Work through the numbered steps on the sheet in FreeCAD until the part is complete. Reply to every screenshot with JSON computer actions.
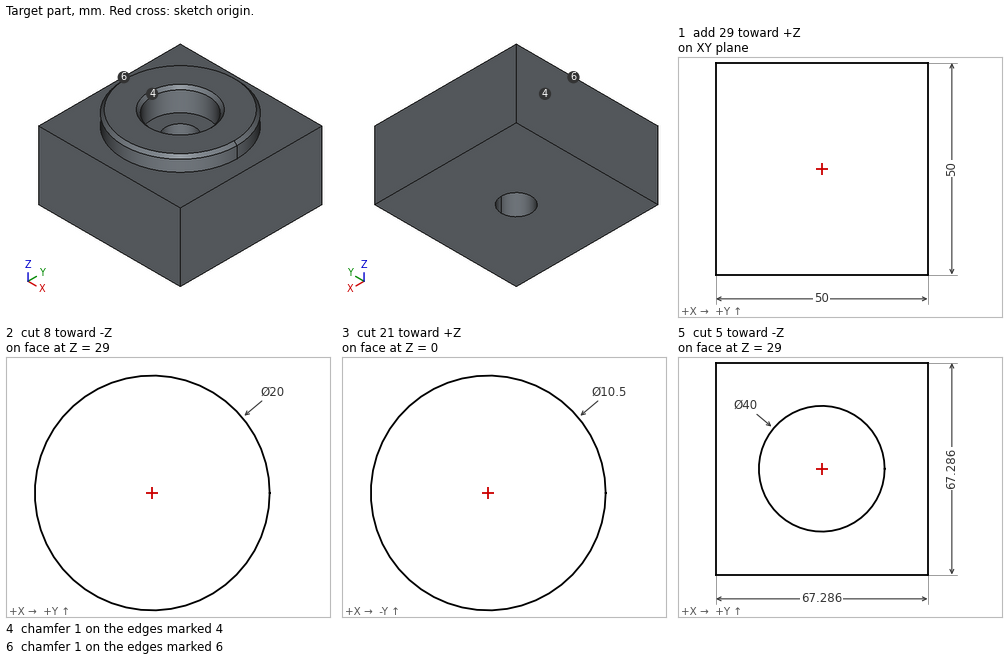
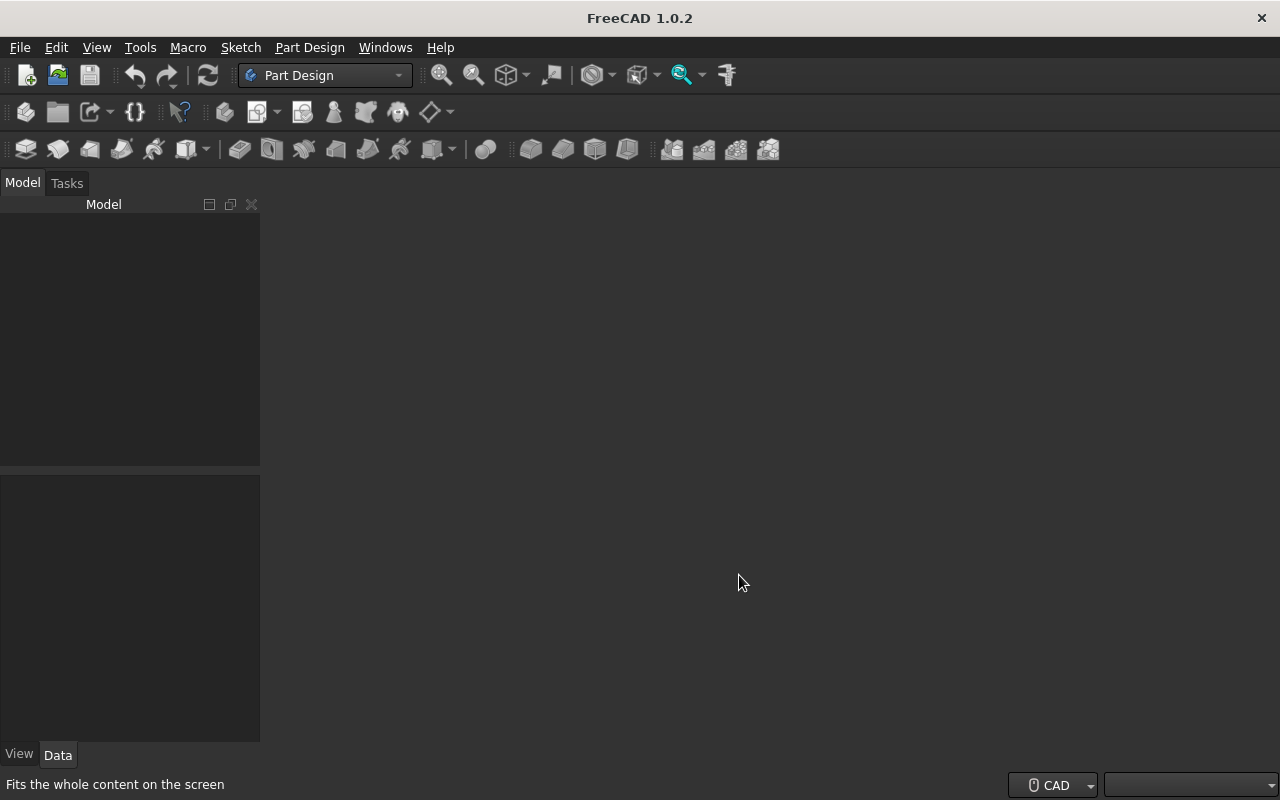
{"action": "left_click", "coordinate": [26, 76]}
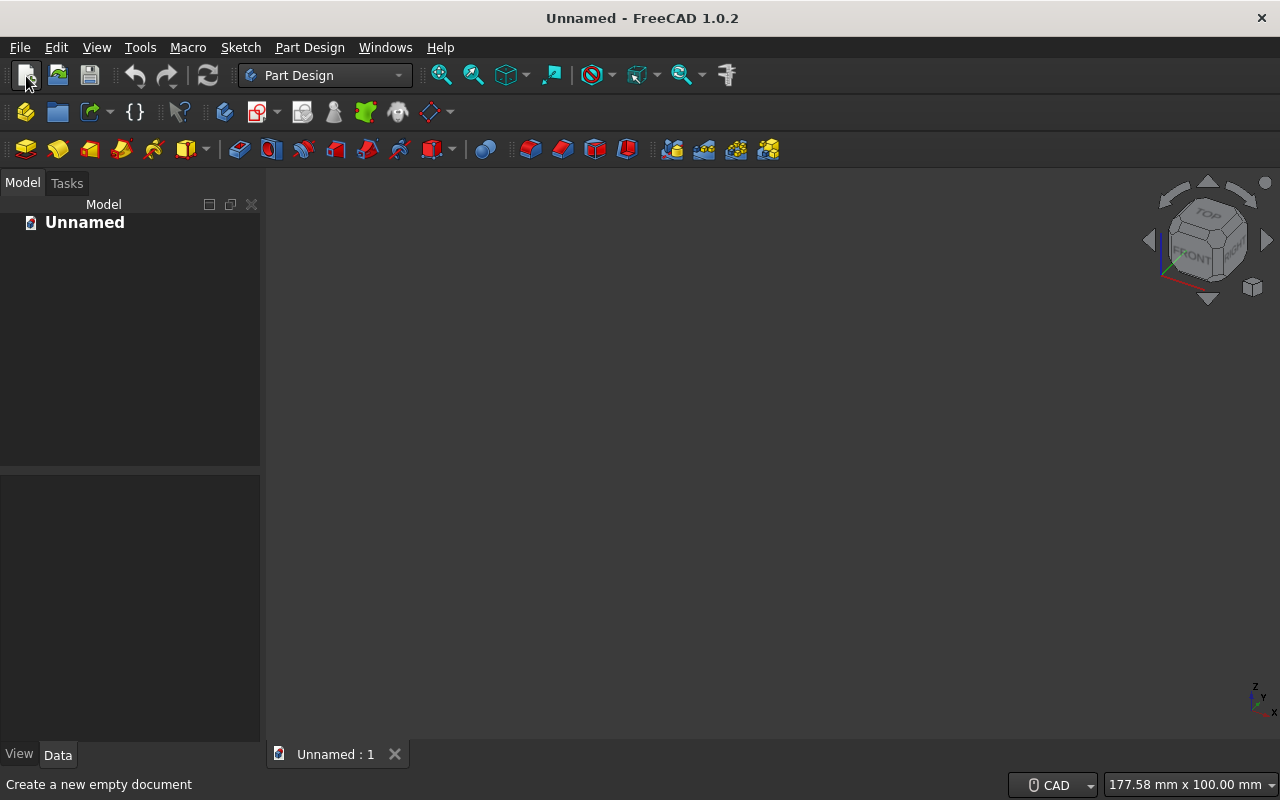
{"action": "left_click", "coordinate": [258, 112]}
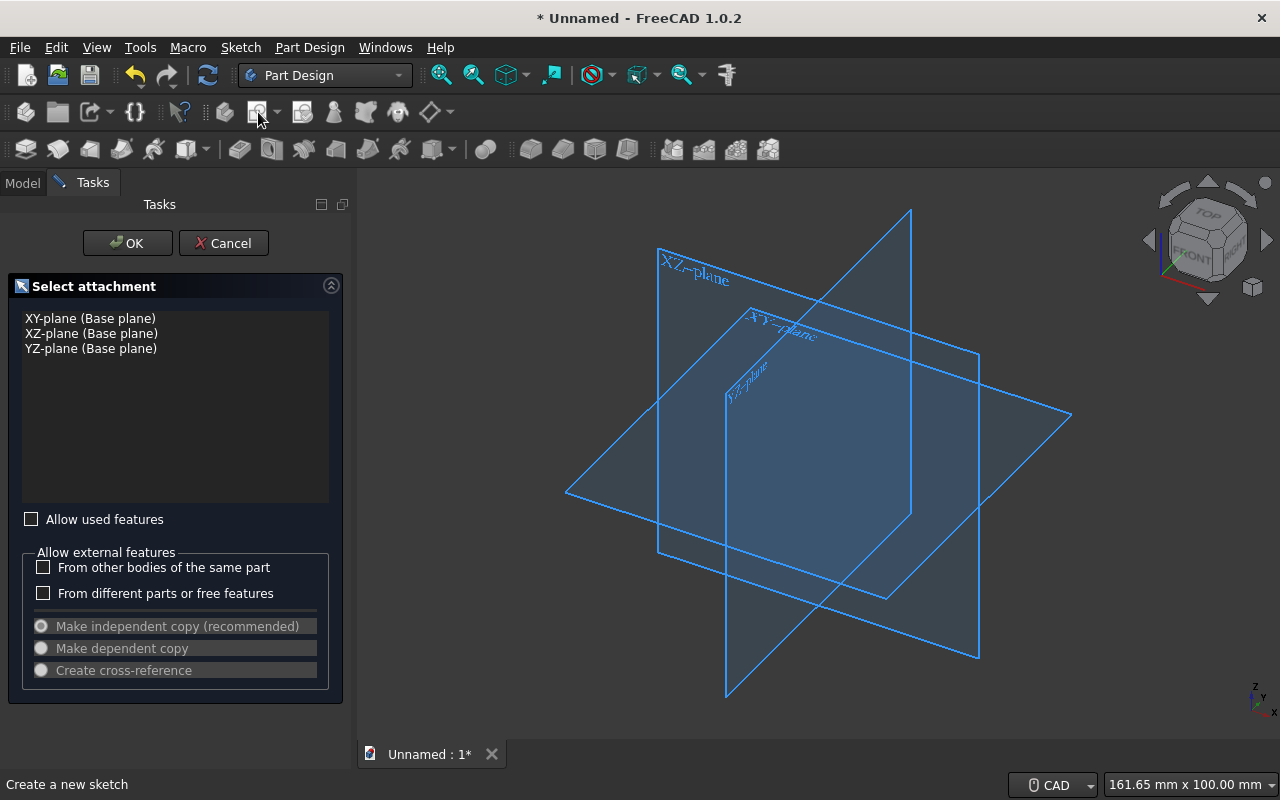
{"action": "left_click", "coordinate": [82, 318]}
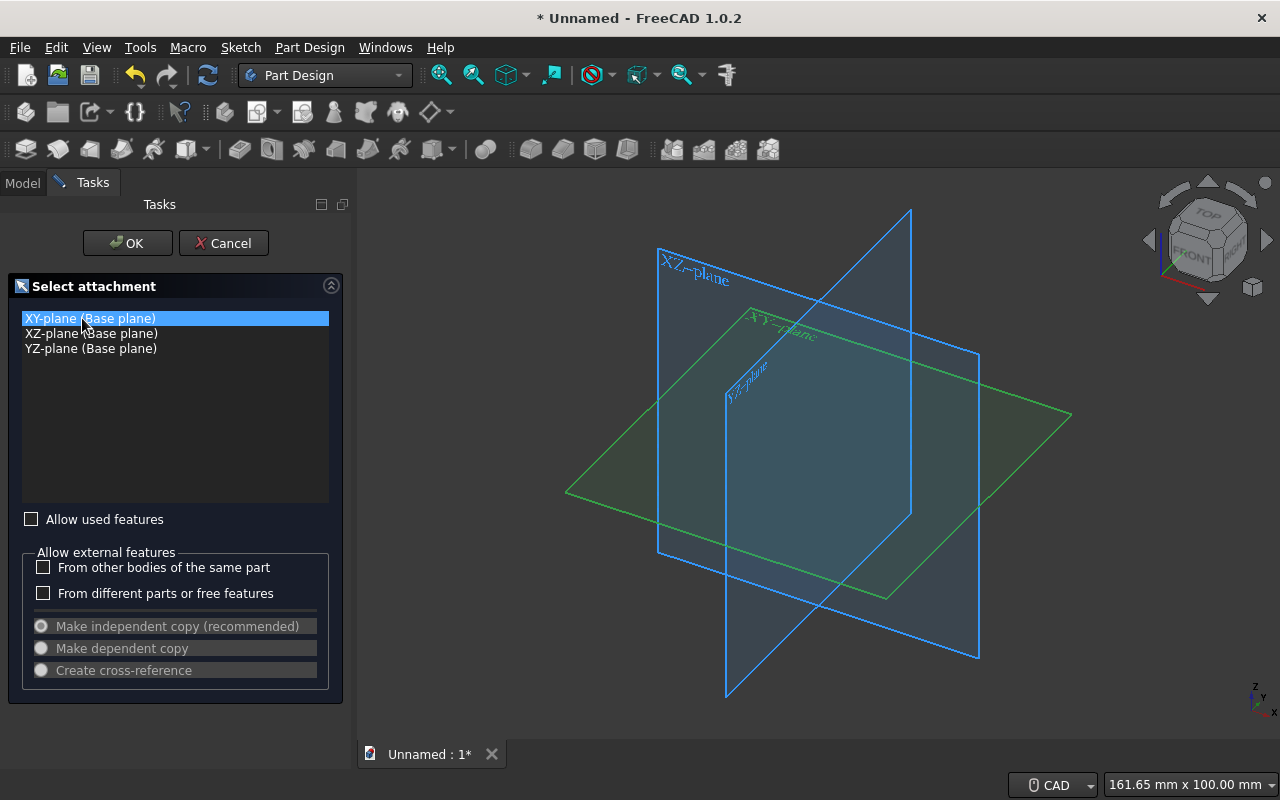
{"action": "left_click", "coordinate": [128, 243]}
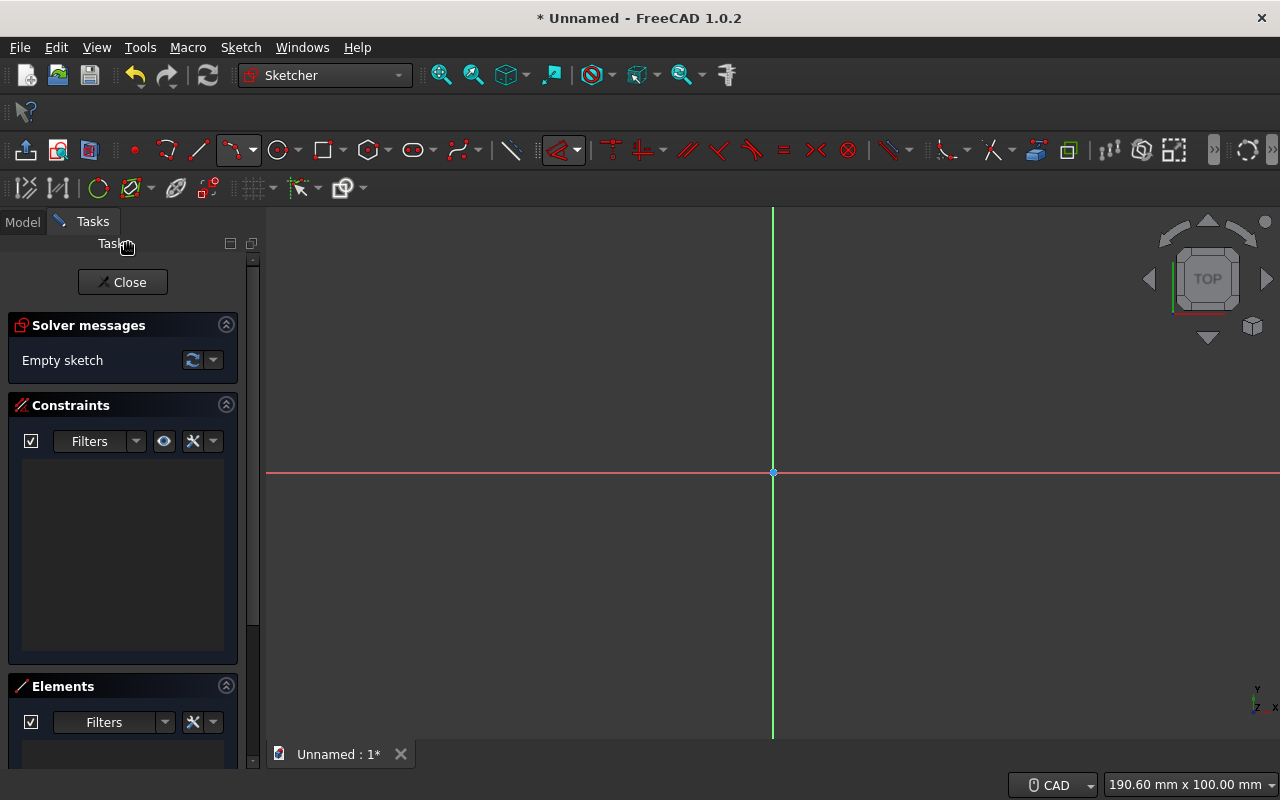
{"action": "key", "text": "g v"}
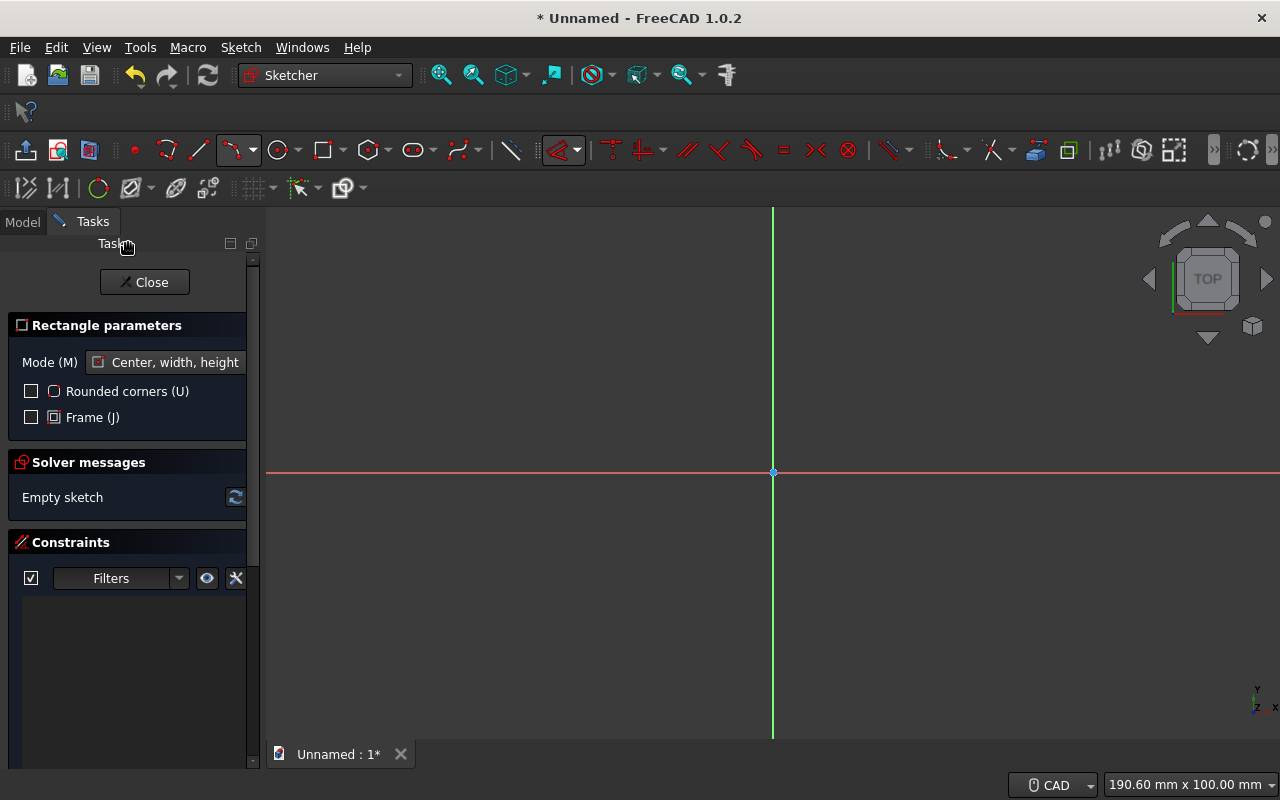
{"action": "left_click", "coordinate": [773, 473]}
{"action": "mouse_move", "coordinate": [906, 340]}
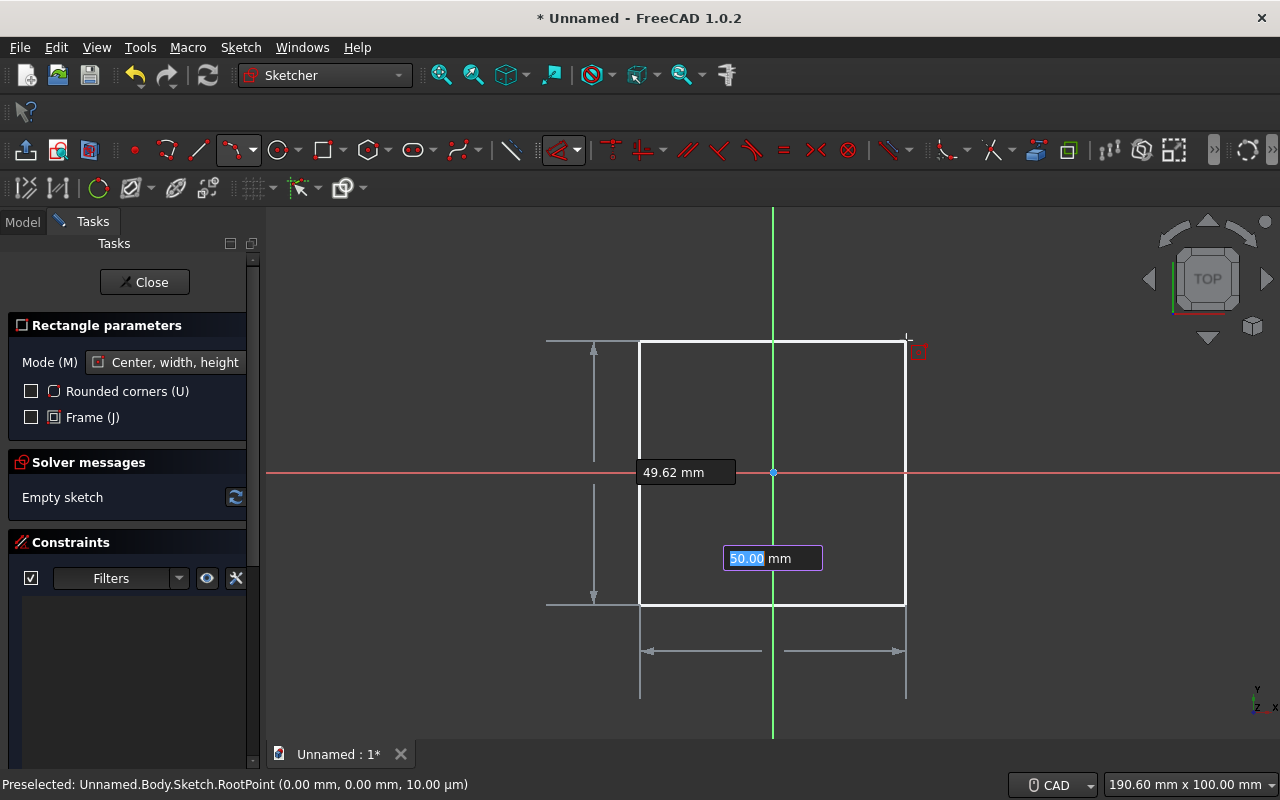
{"action": "type", "text": "50"}
{"action": "key", "text": "Tab"}
{"action": "type", "text": "50"}
{"action": "key", "text": "Return"}
{"action": "key", "text": "Escape"}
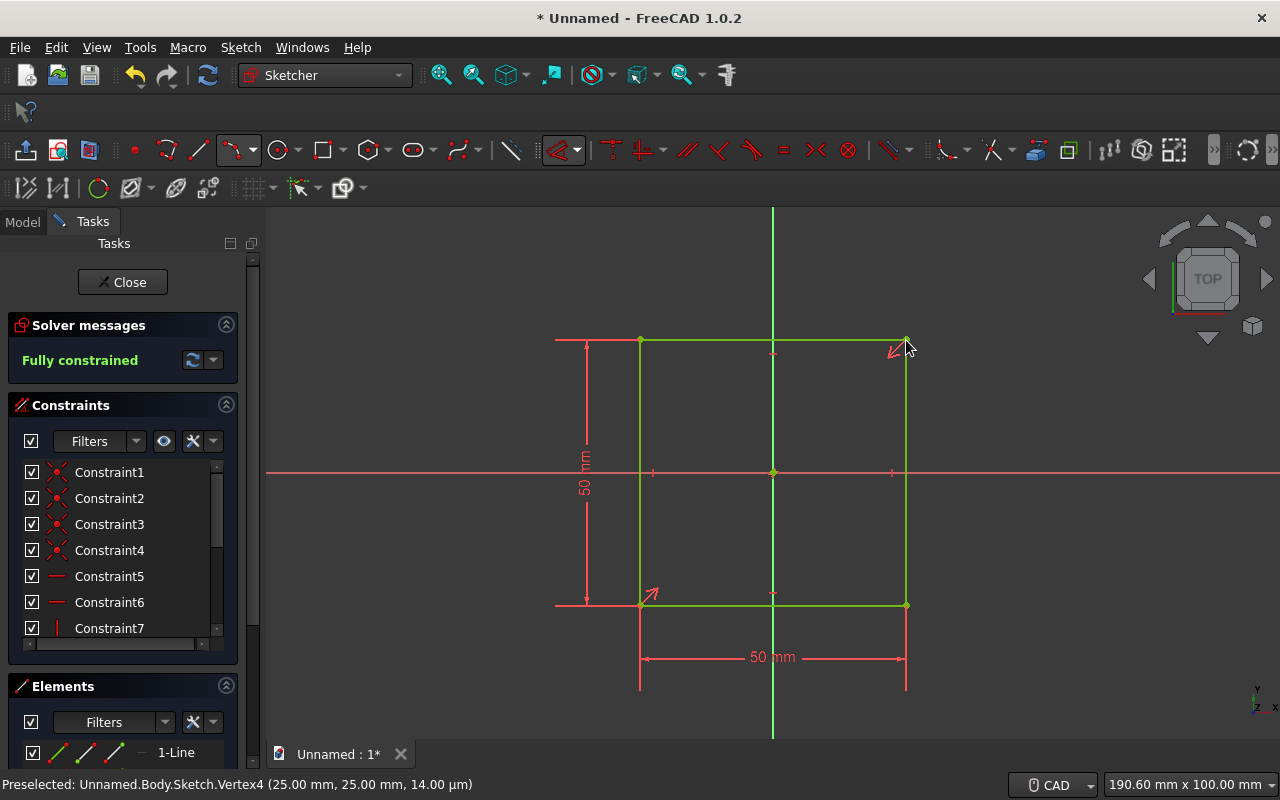
{"action": "left_click", "coordinate": [123, 282]}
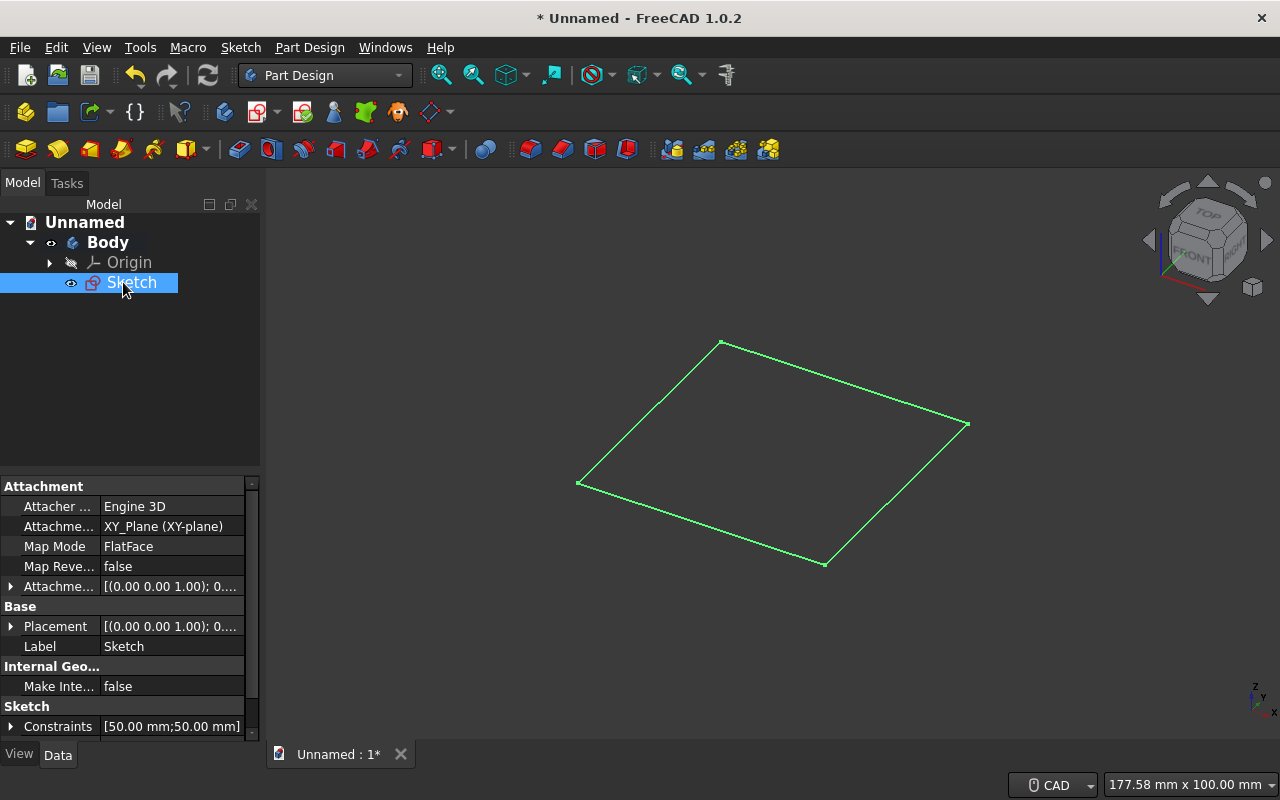
{"action": "left_click", "coordinate": [26, 150]}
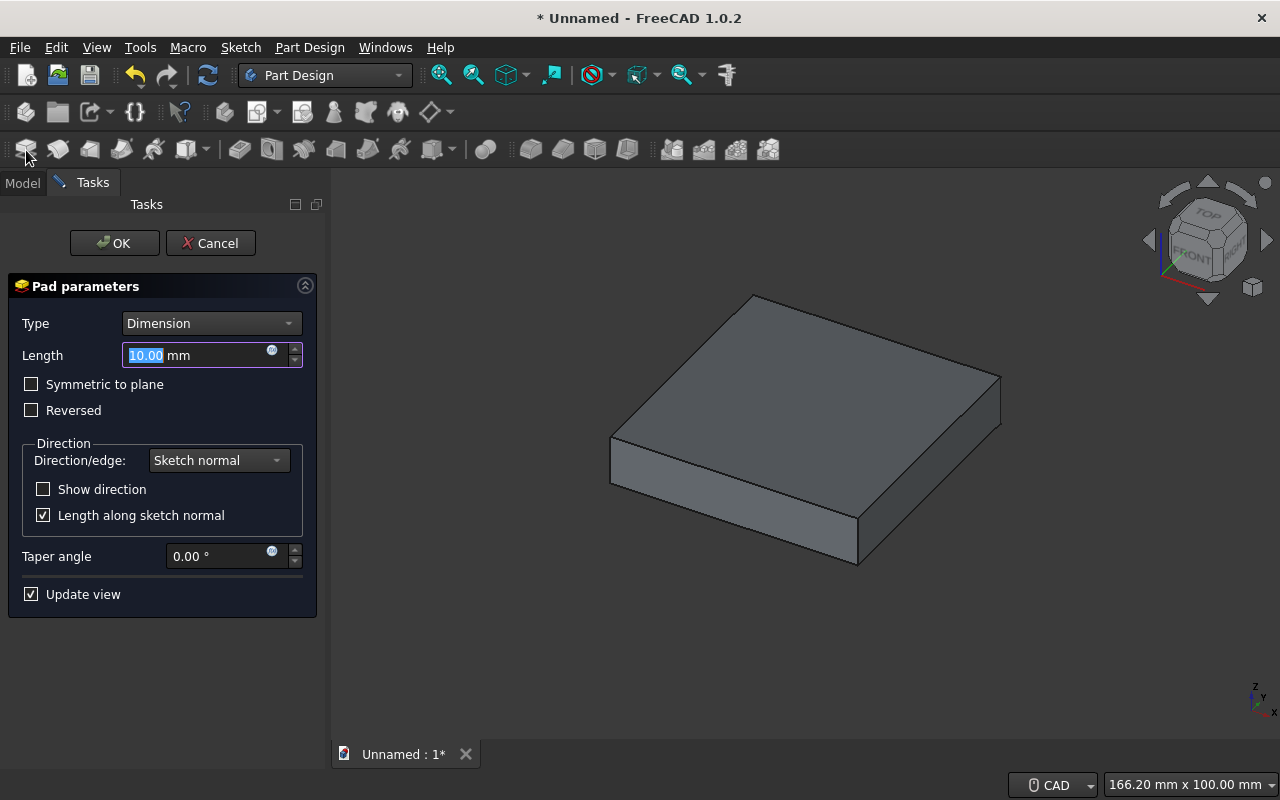
{"action": "type", "text": "29"}
{"action": "key", "text": "Tab"}